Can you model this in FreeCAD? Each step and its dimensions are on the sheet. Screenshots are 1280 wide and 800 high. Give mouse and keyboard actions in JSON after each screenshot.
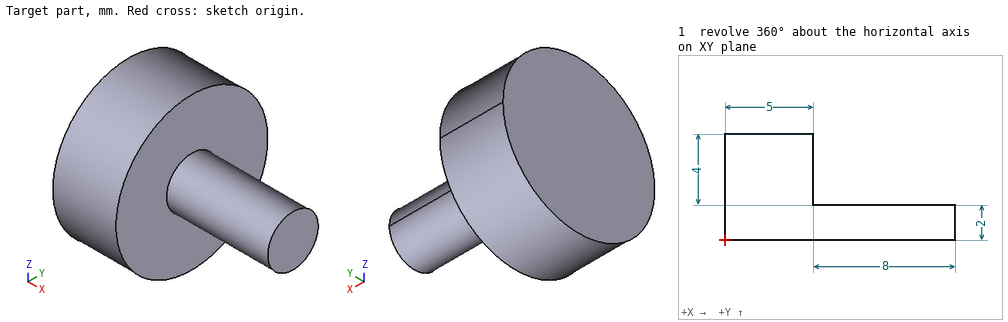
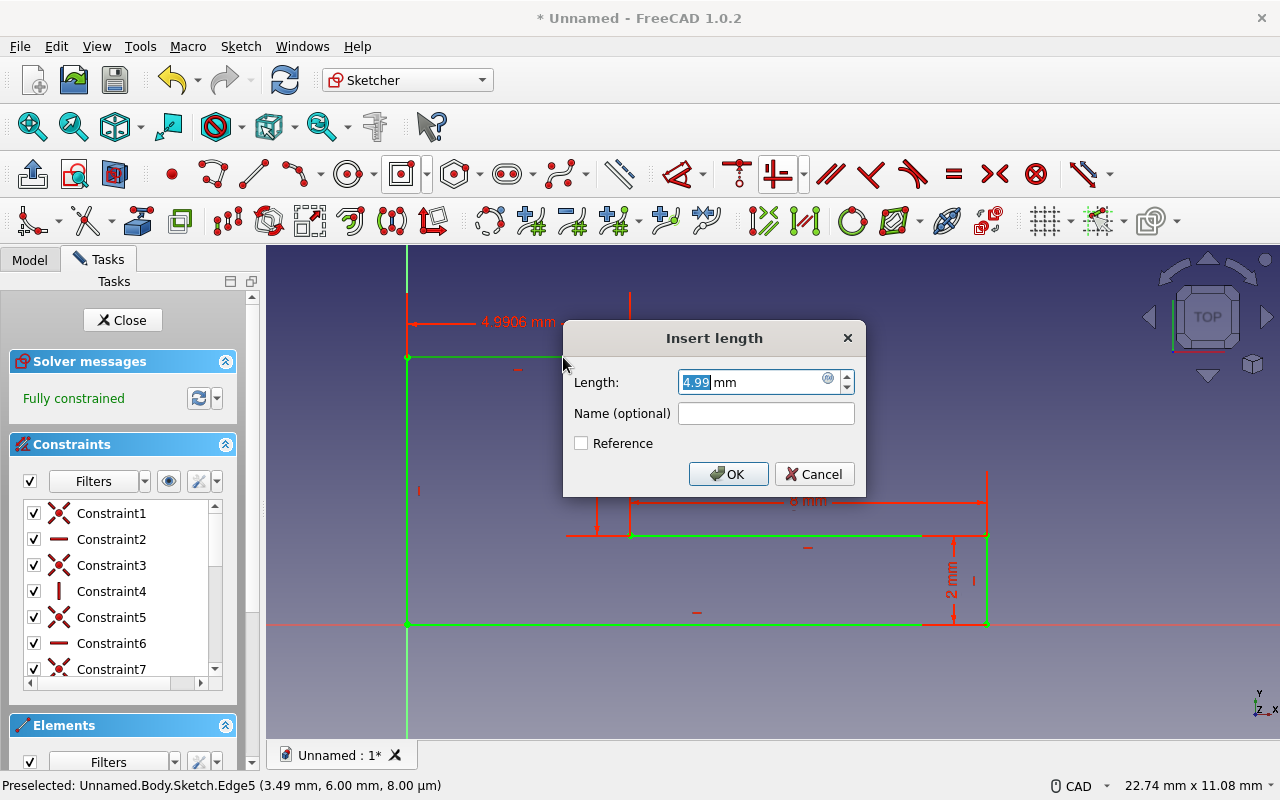
{"action": "type", "text": "5"}
{"action": "key", "text": "Return"}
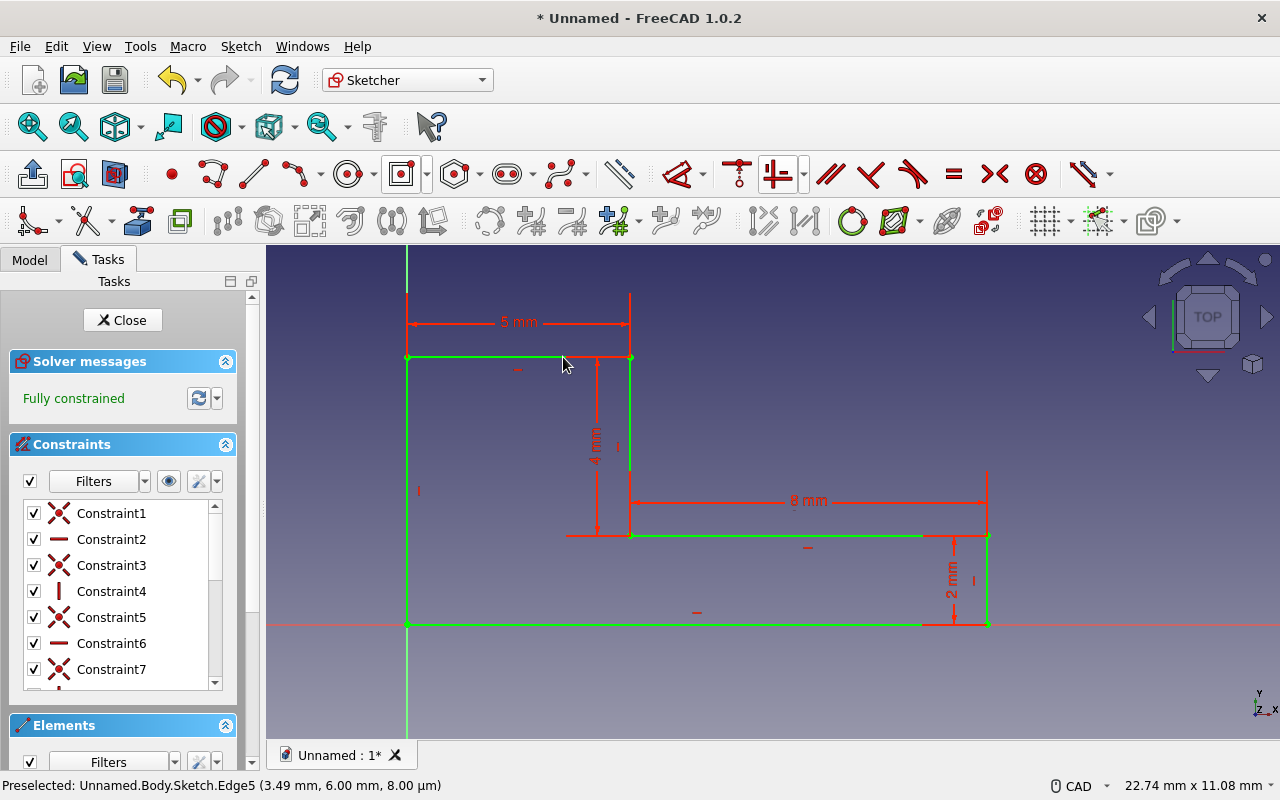
{"action": "left_click", "coordinate": [123, 320]}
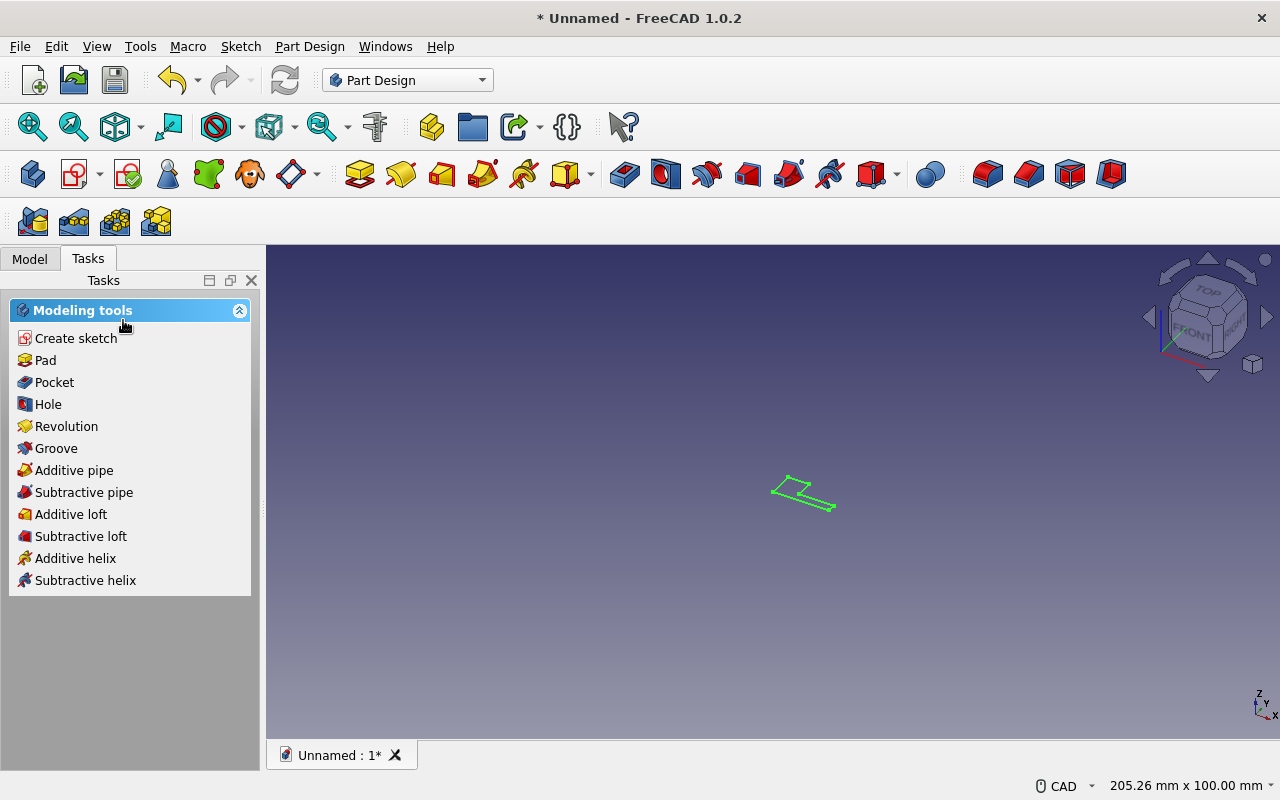
{"action": "left_click", "coordinate": [401, 174]}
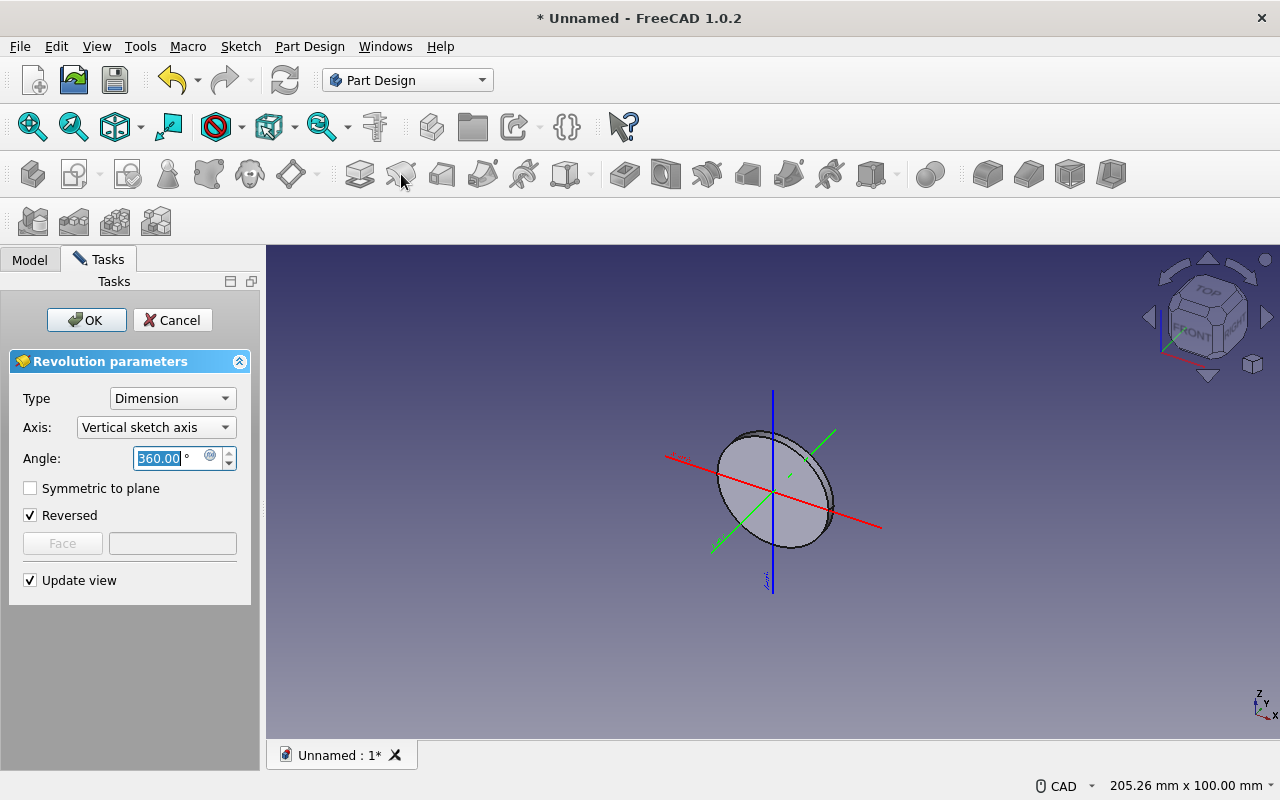
{"action": "left_click", "coordinate": [157, 428]}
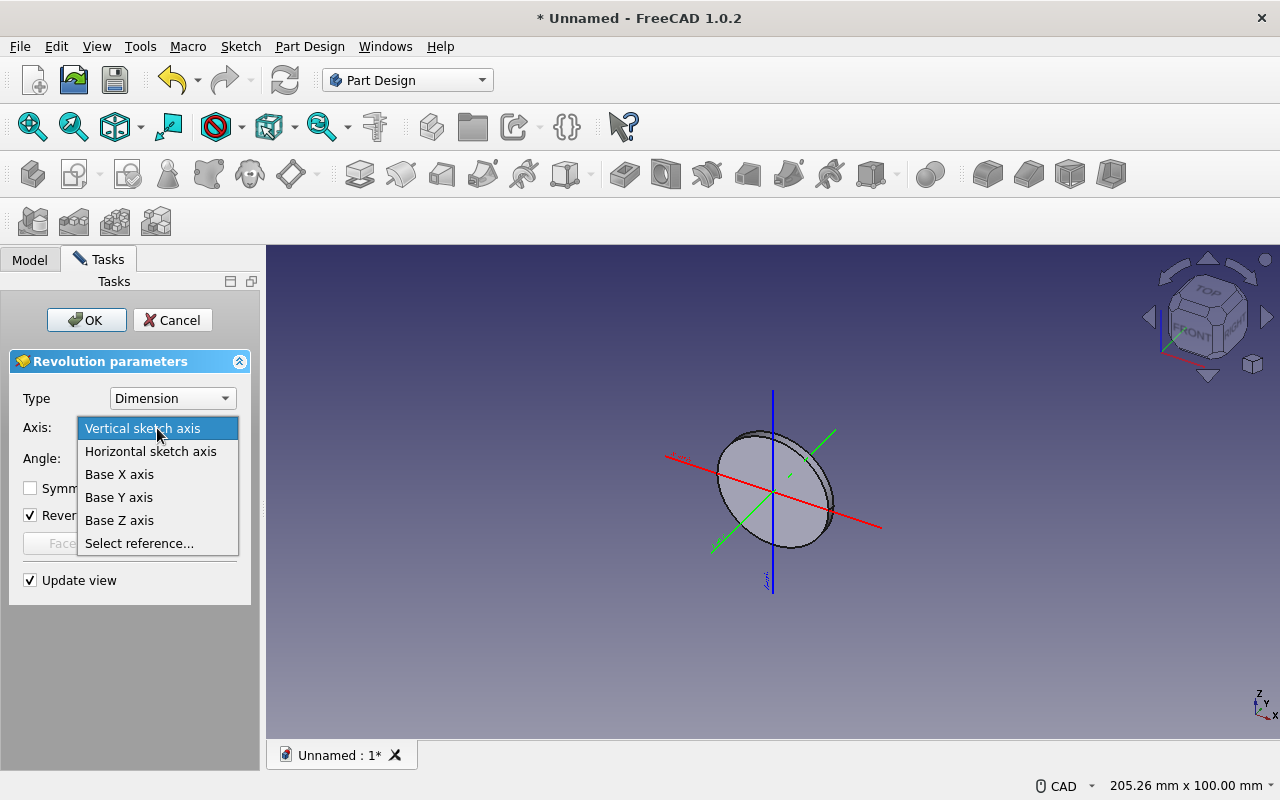
{"action": "left_click", "coordinate": [156, 452]}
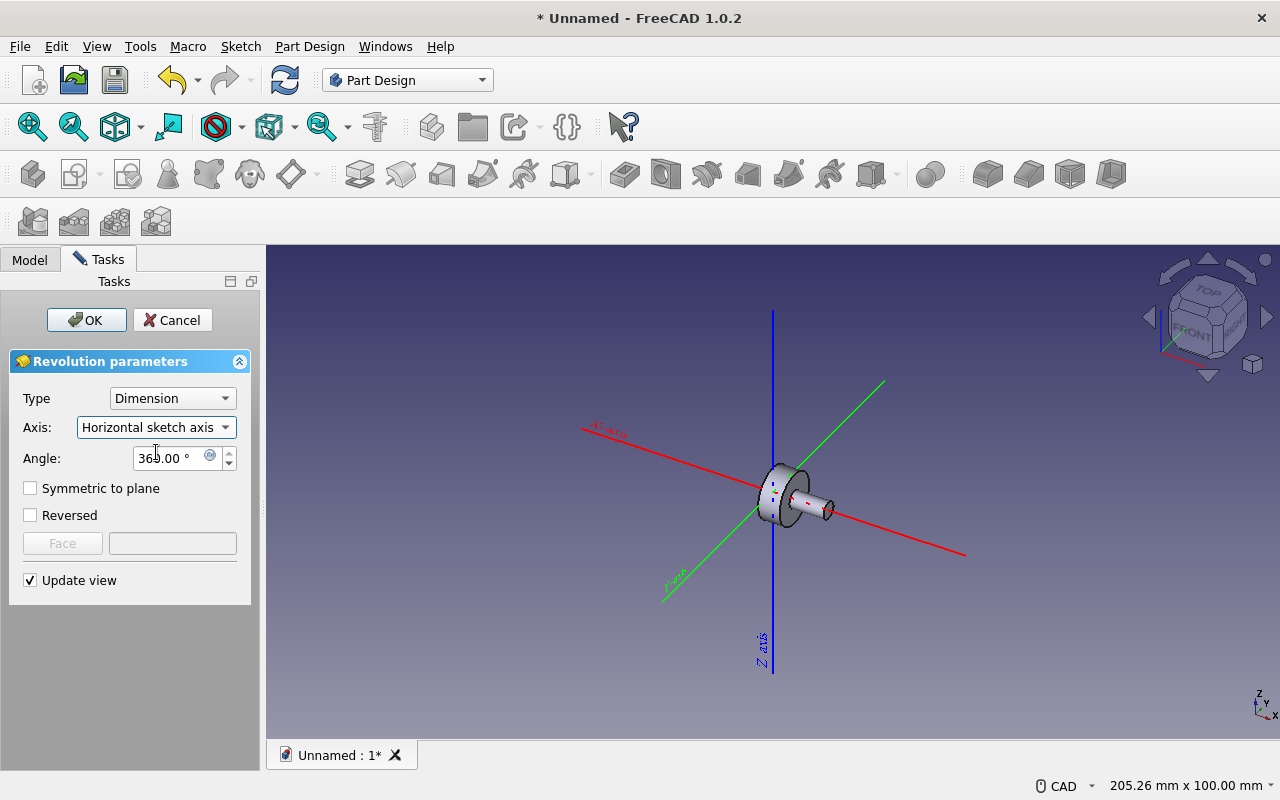
{"action": "left_click", "coordinate": [87, 320]}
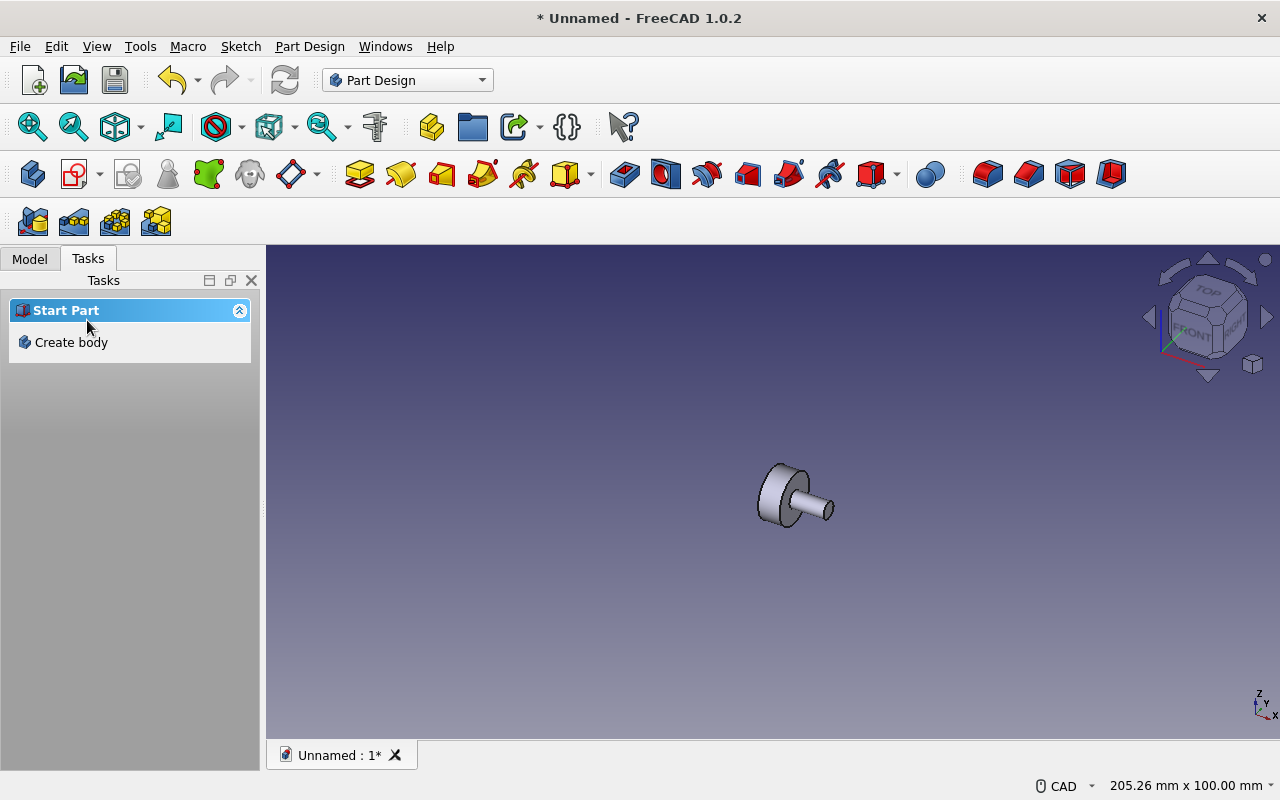
{"action": "key", "text": "0"}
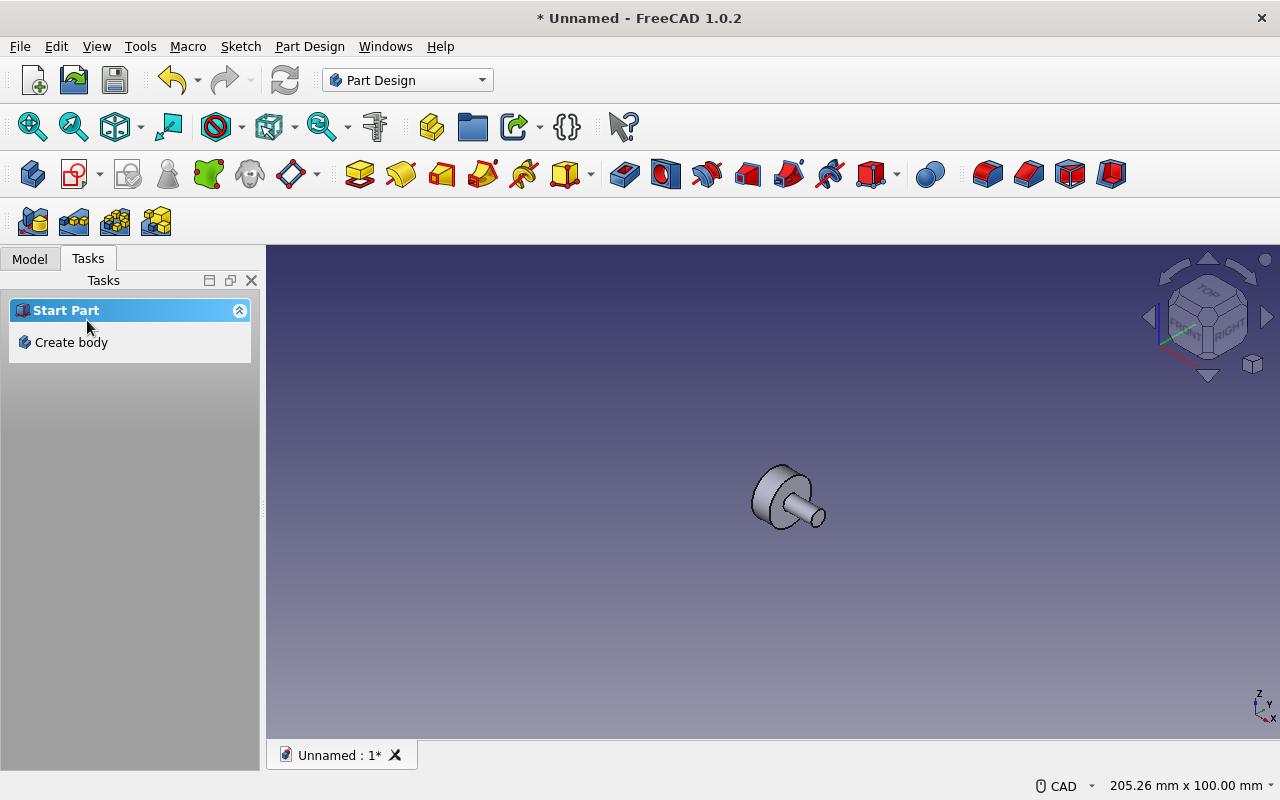
{"action": "left_click", "coordinate": [33, 128]}